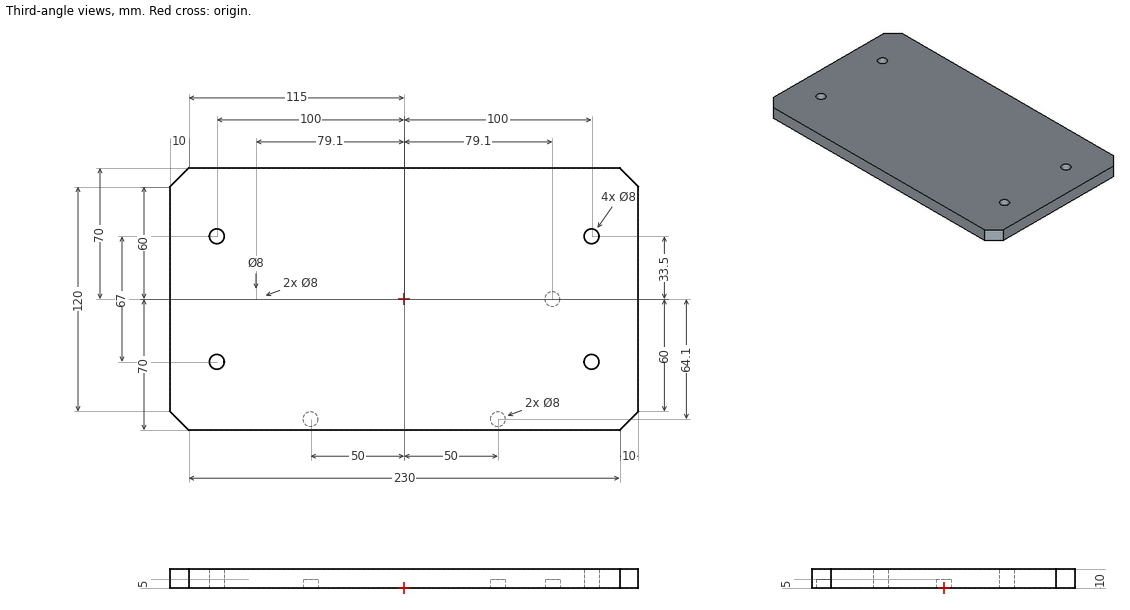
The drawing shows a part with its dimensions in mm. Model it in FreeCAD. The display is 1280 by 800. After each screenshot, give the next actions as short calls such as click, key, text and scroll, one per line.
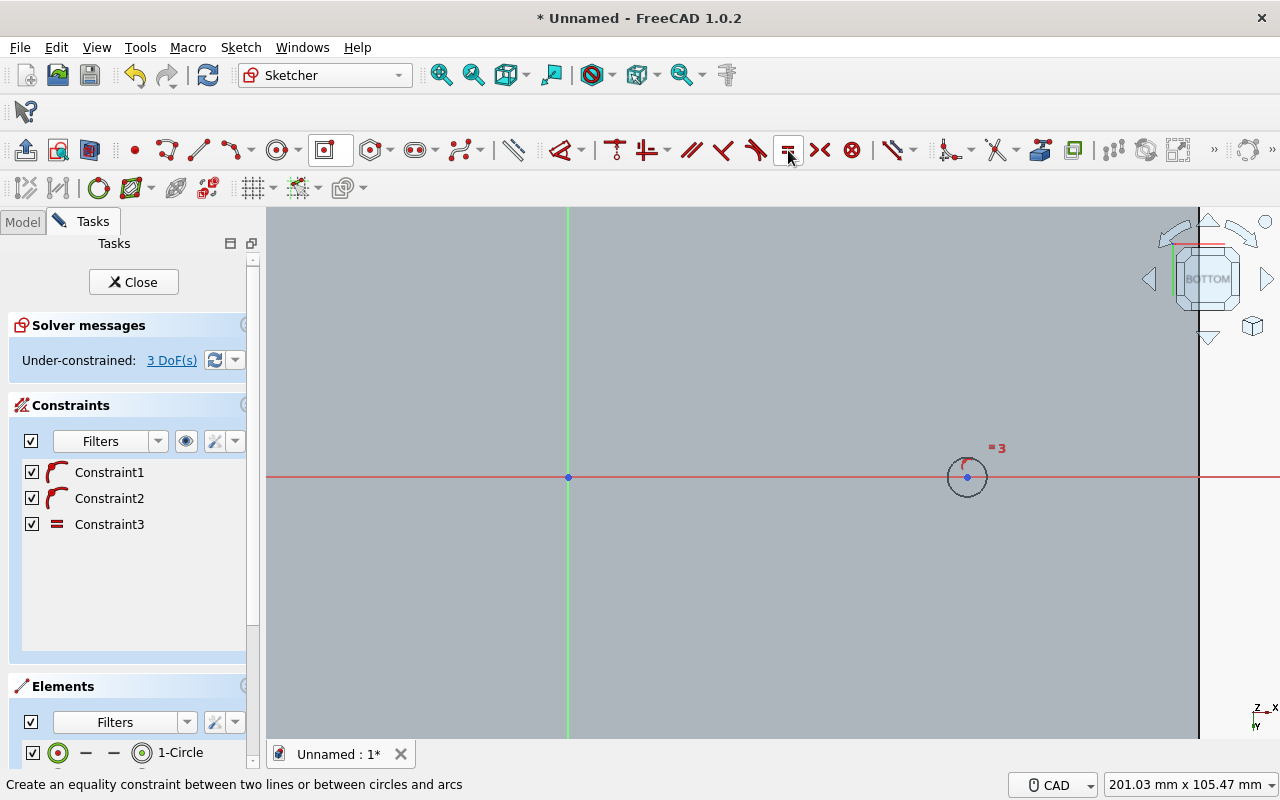
click(560, 150)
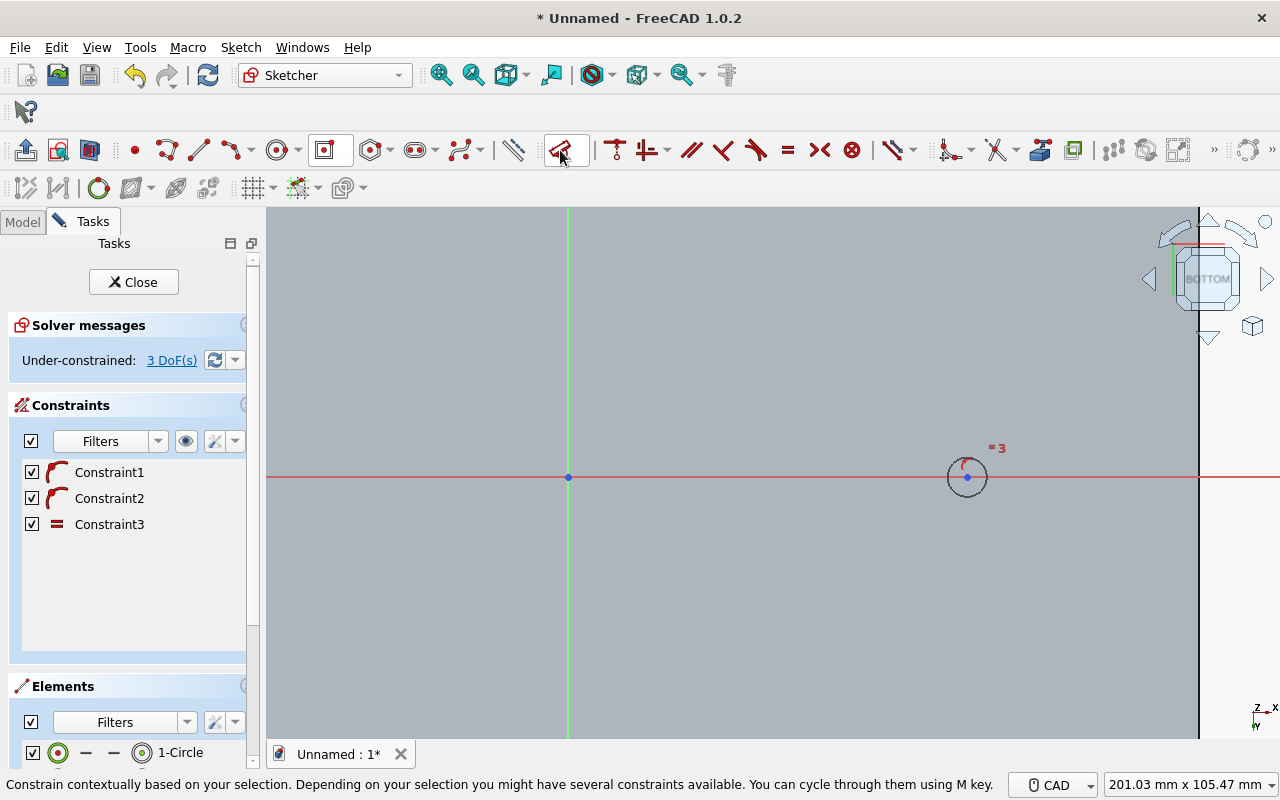
scroll(982, 464, down, 2)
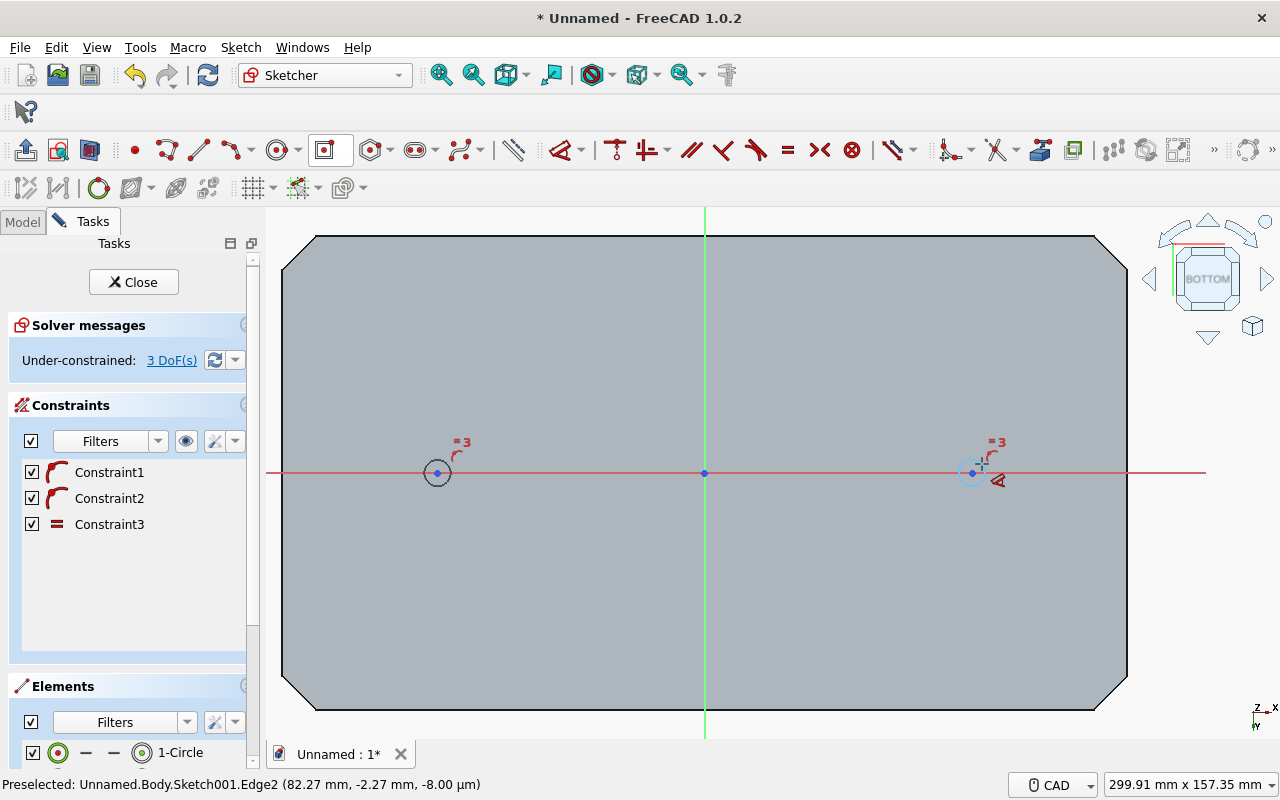
scroll(447, 464, up, 2)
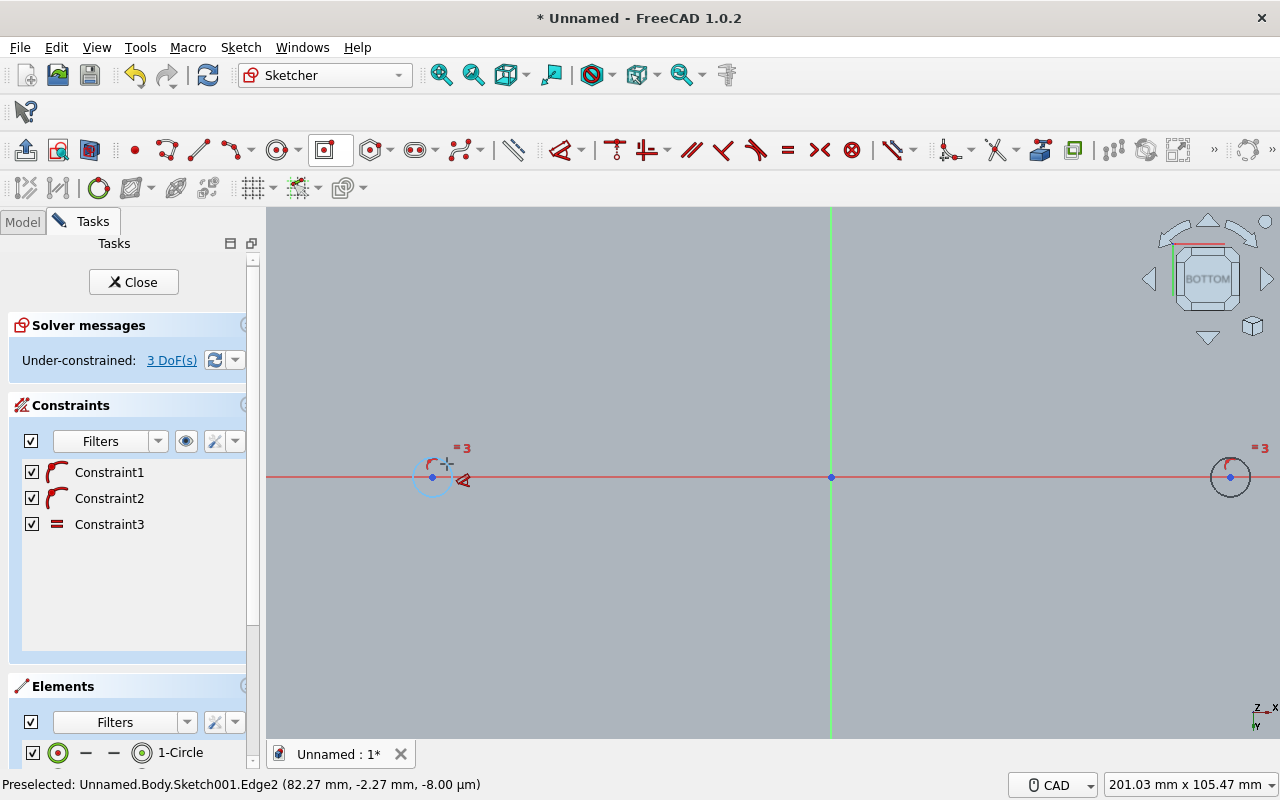
click(447, 463)
click(470, 440)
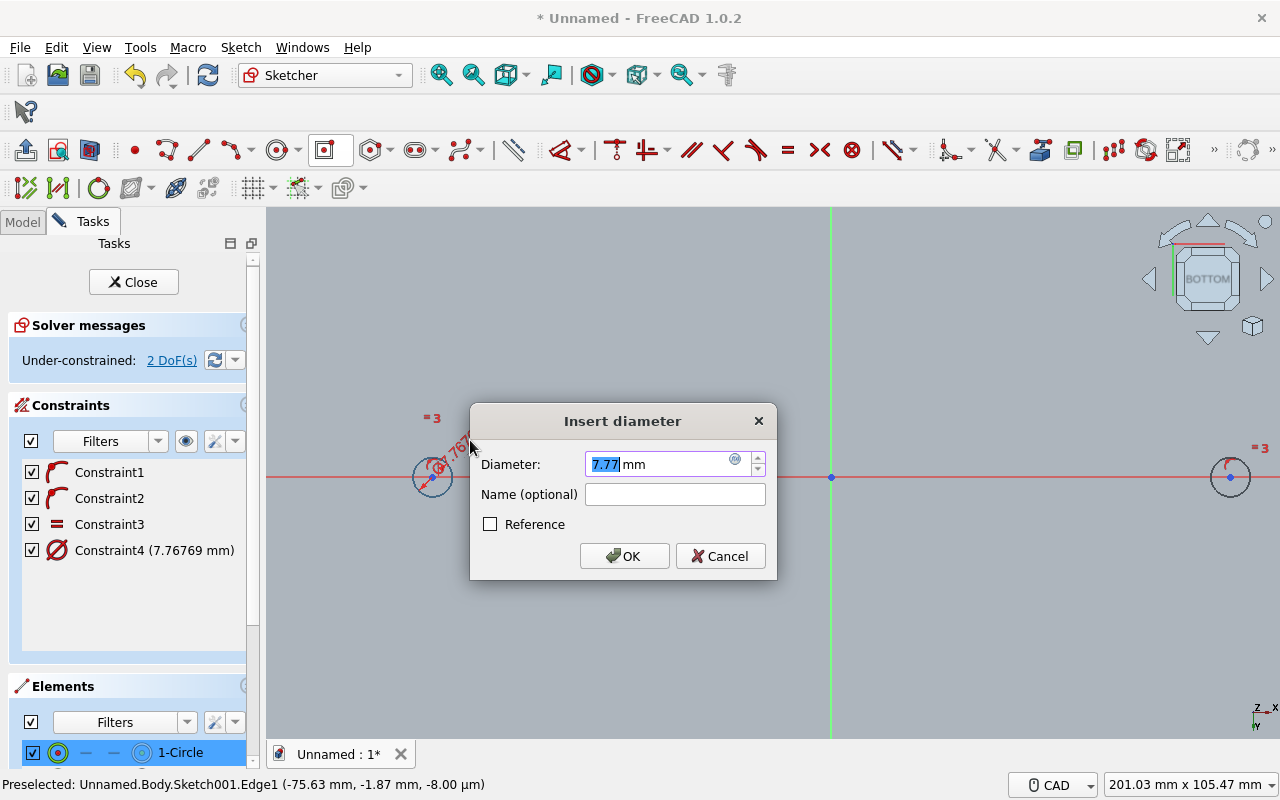
text(8)
key(Return)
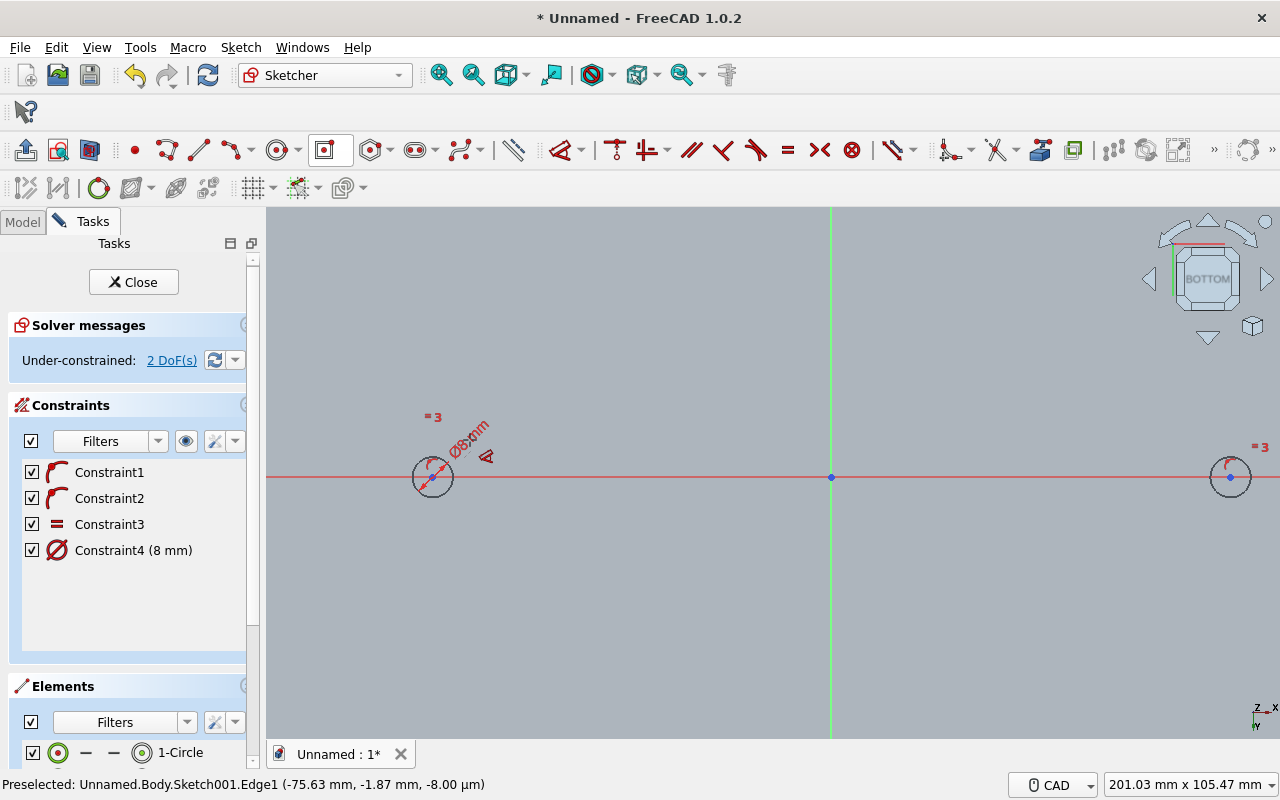
click(433, 477)
click(632, 511)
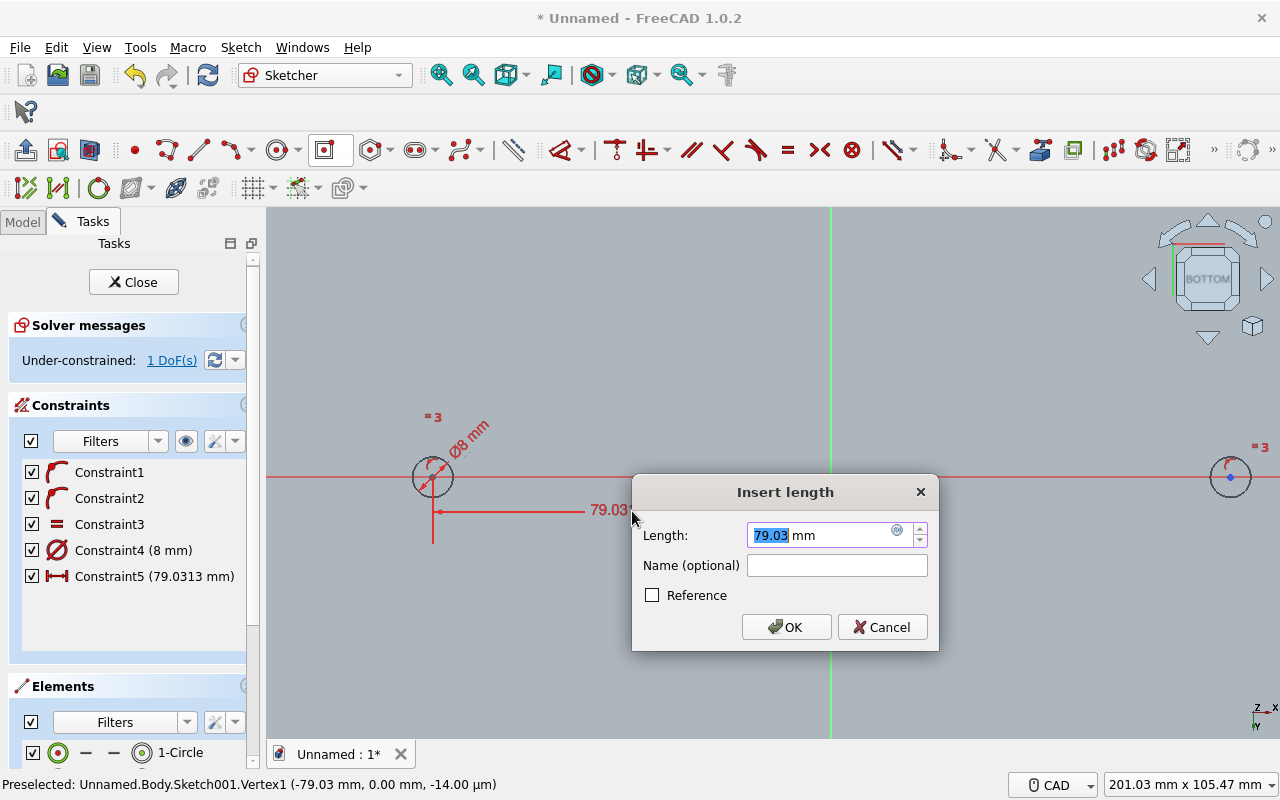
text(79.1)
key(Return)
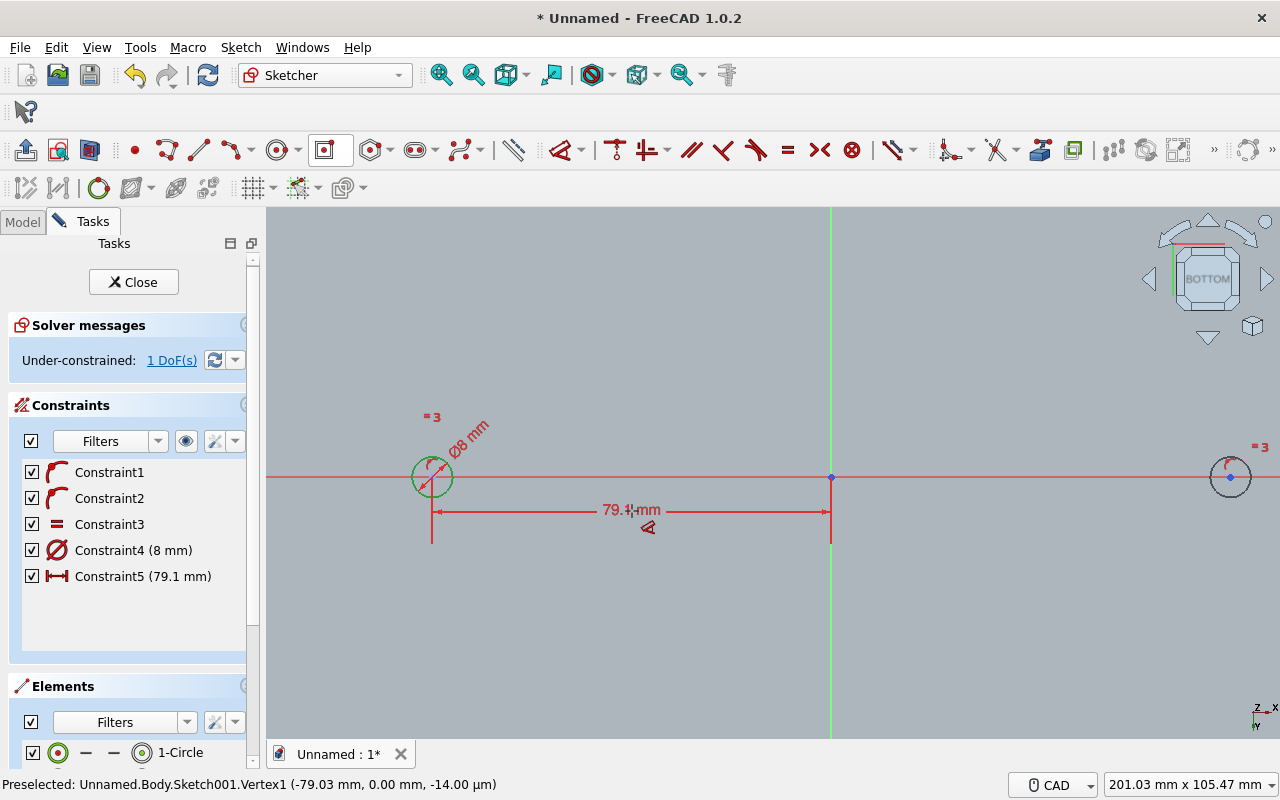
scroll(446, 464, down, 2)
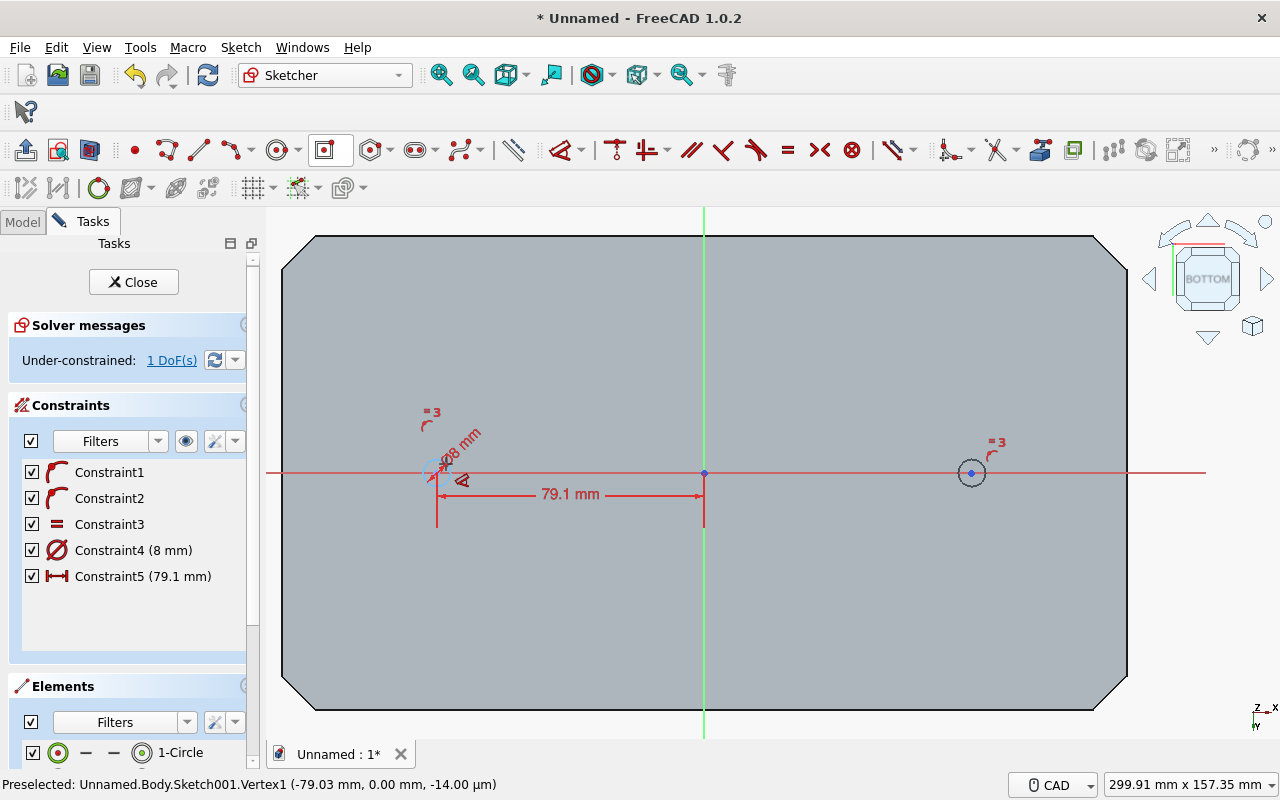
click(972, 473)
click(838, 507)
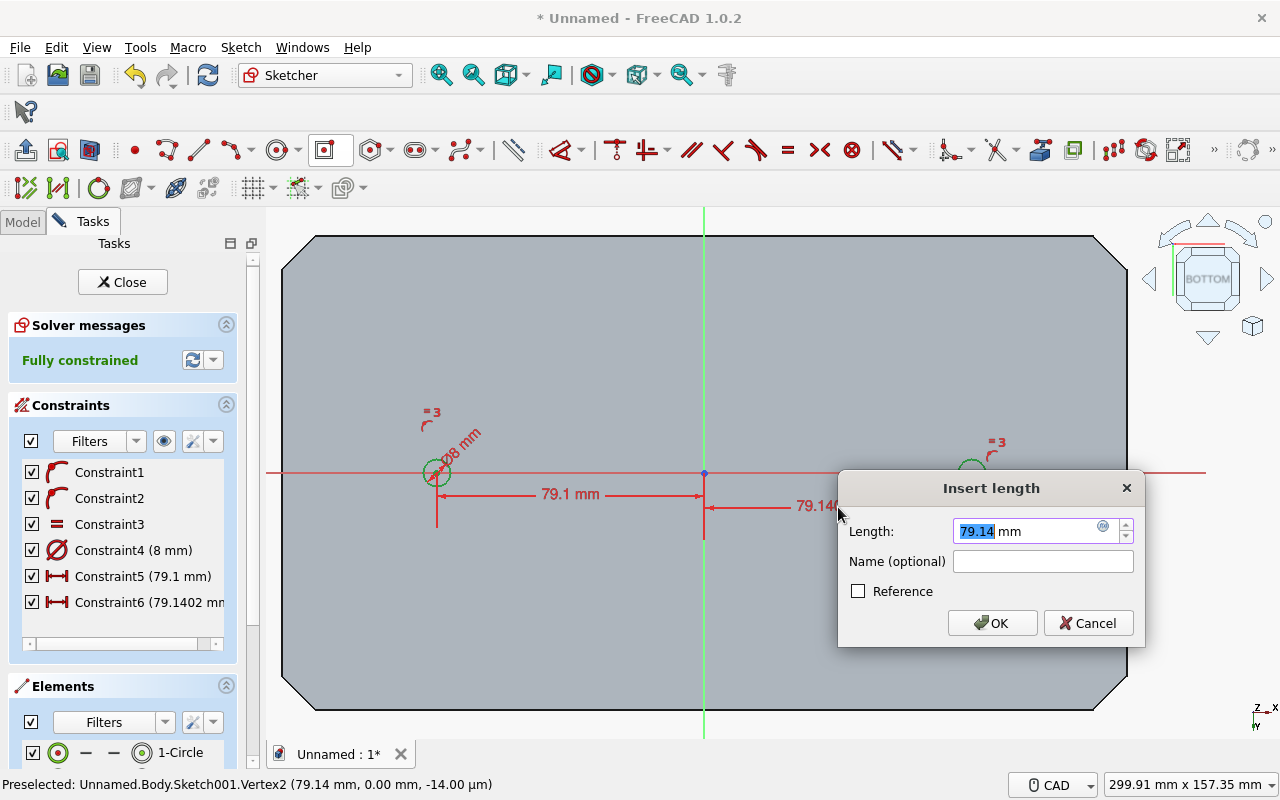
text(79.1)
key(Return)
key(Escape)